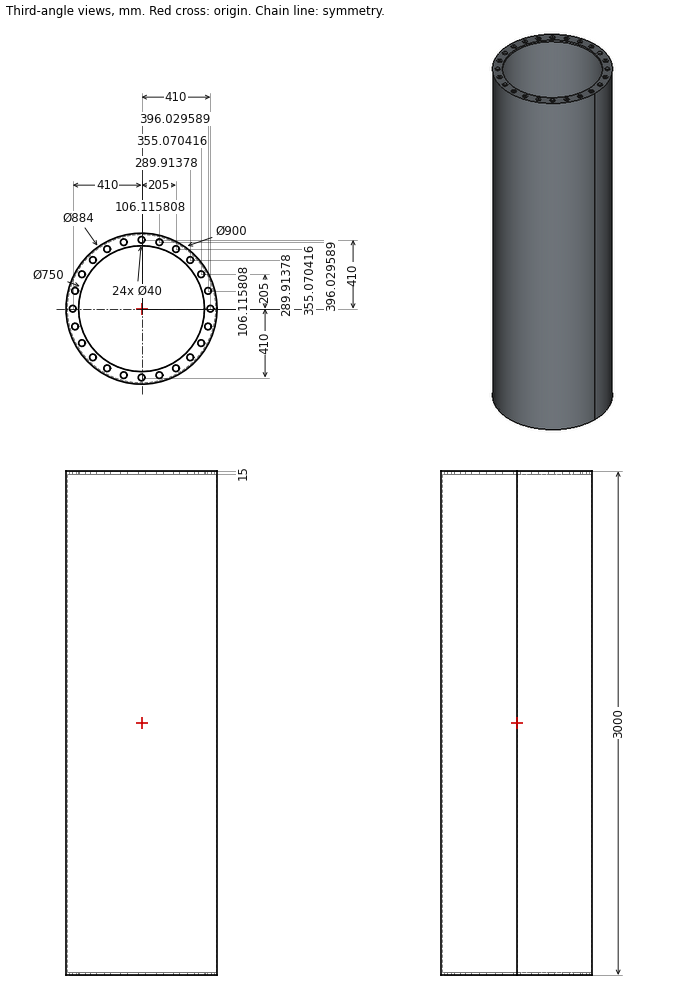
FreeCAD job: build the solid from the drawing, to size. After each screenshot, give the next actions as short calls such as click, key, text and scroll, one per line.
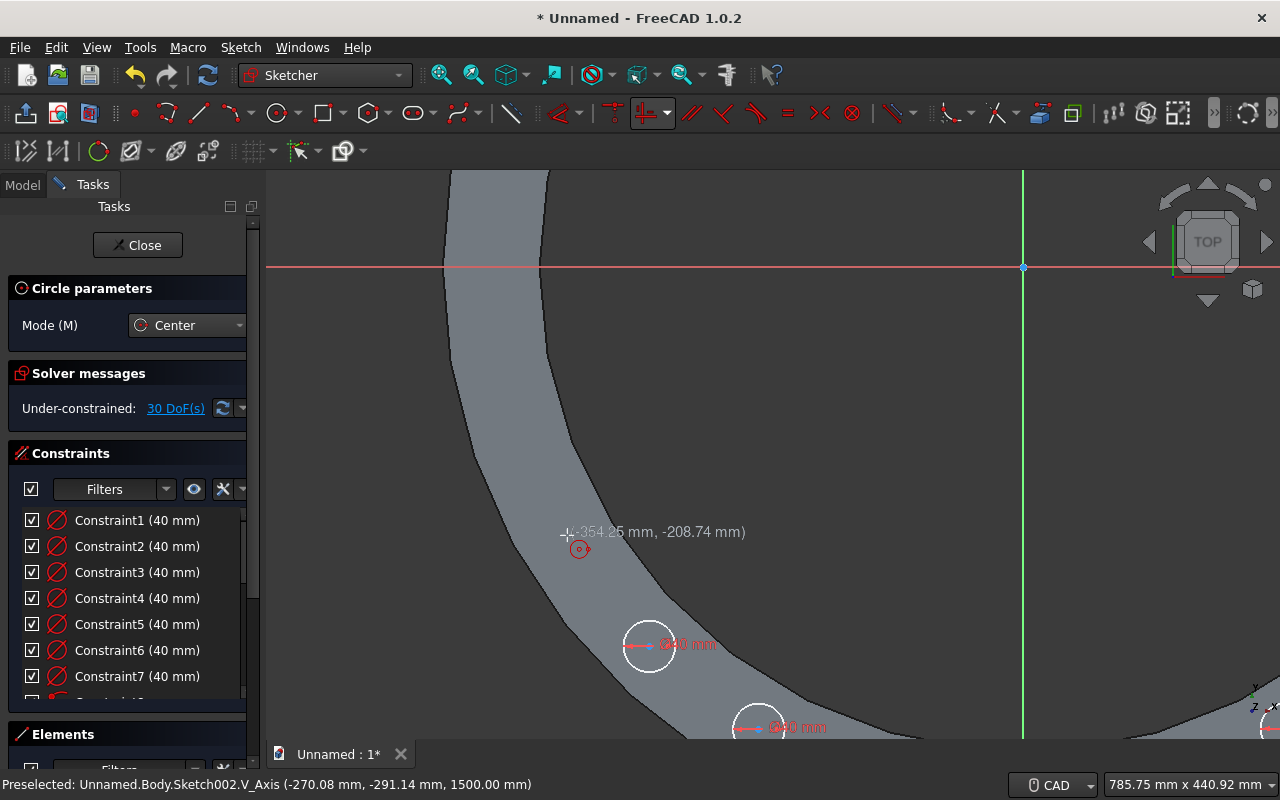
scroll(567, 535, down, 6)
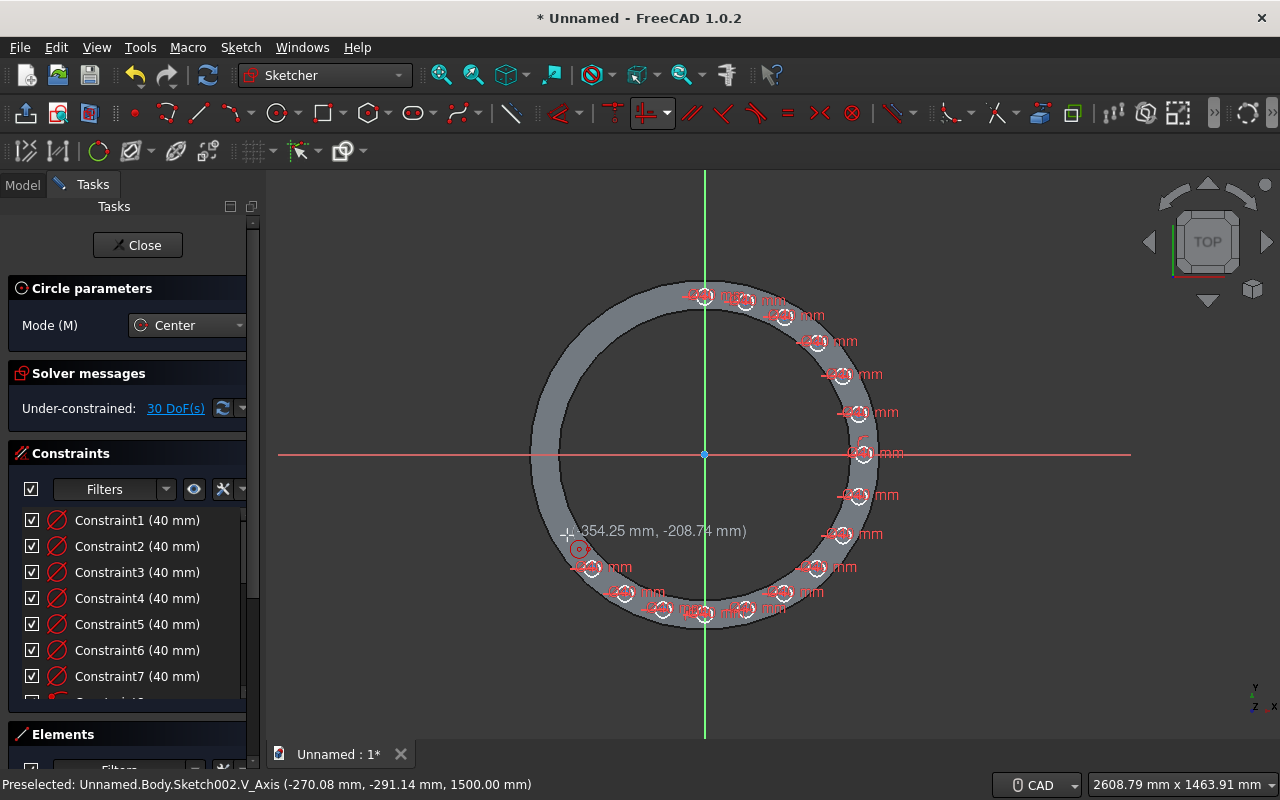
click(567, 535)
move(572, 529)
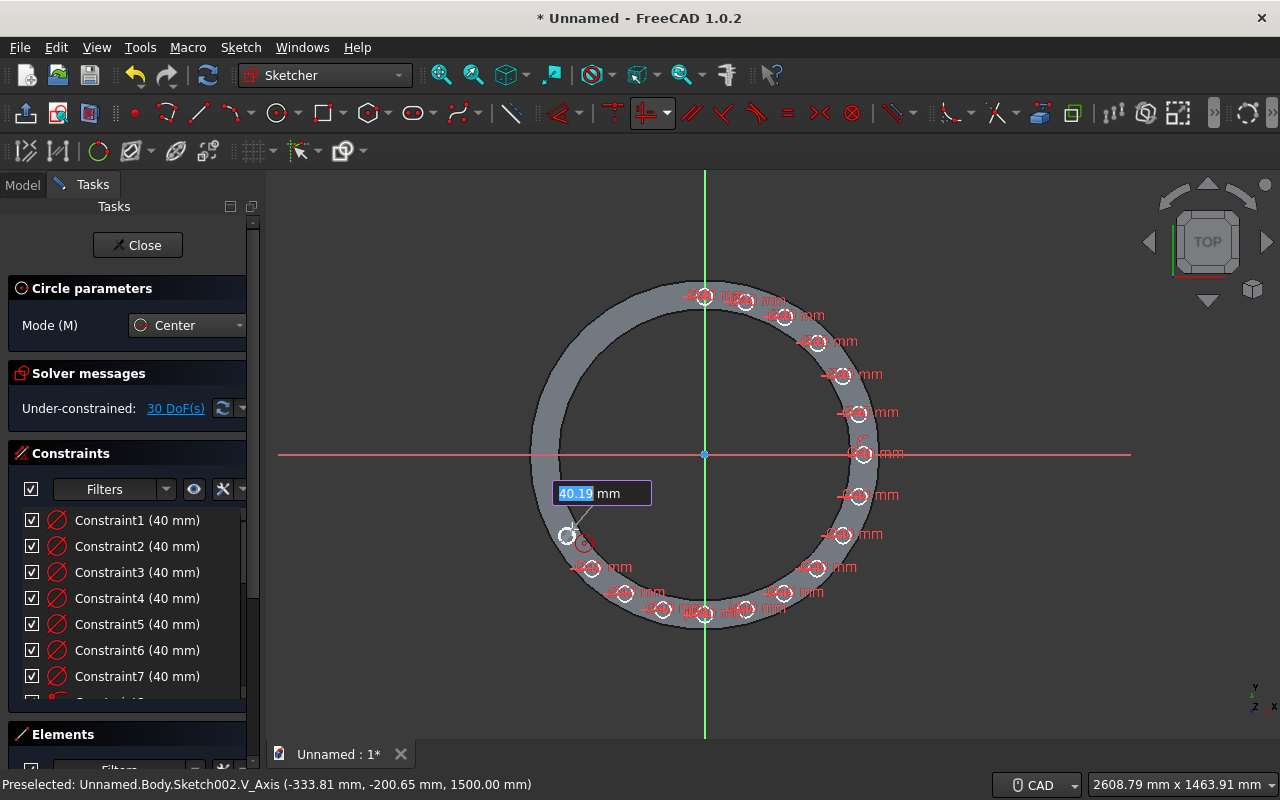
text(40)
key(Return)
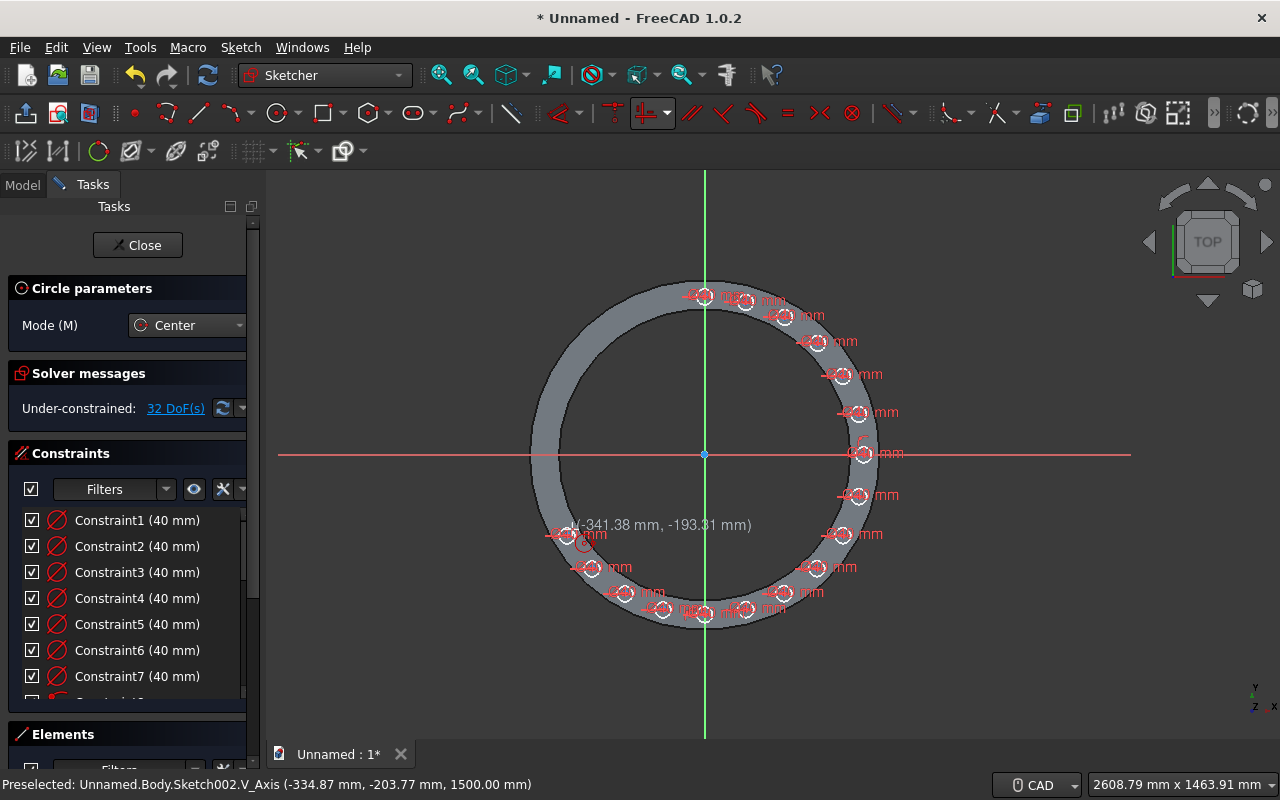
scroll(551, 496, up, 6)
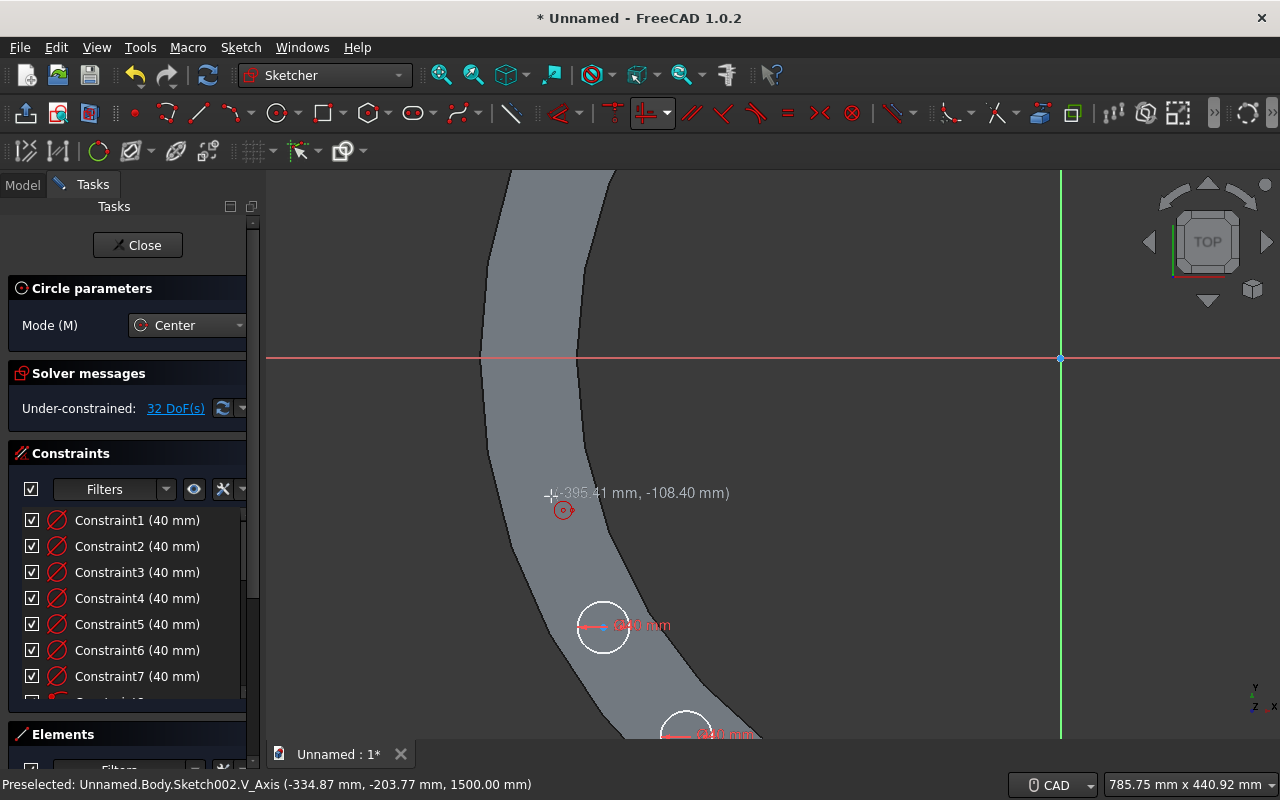
scroll(551, 496, down, 6)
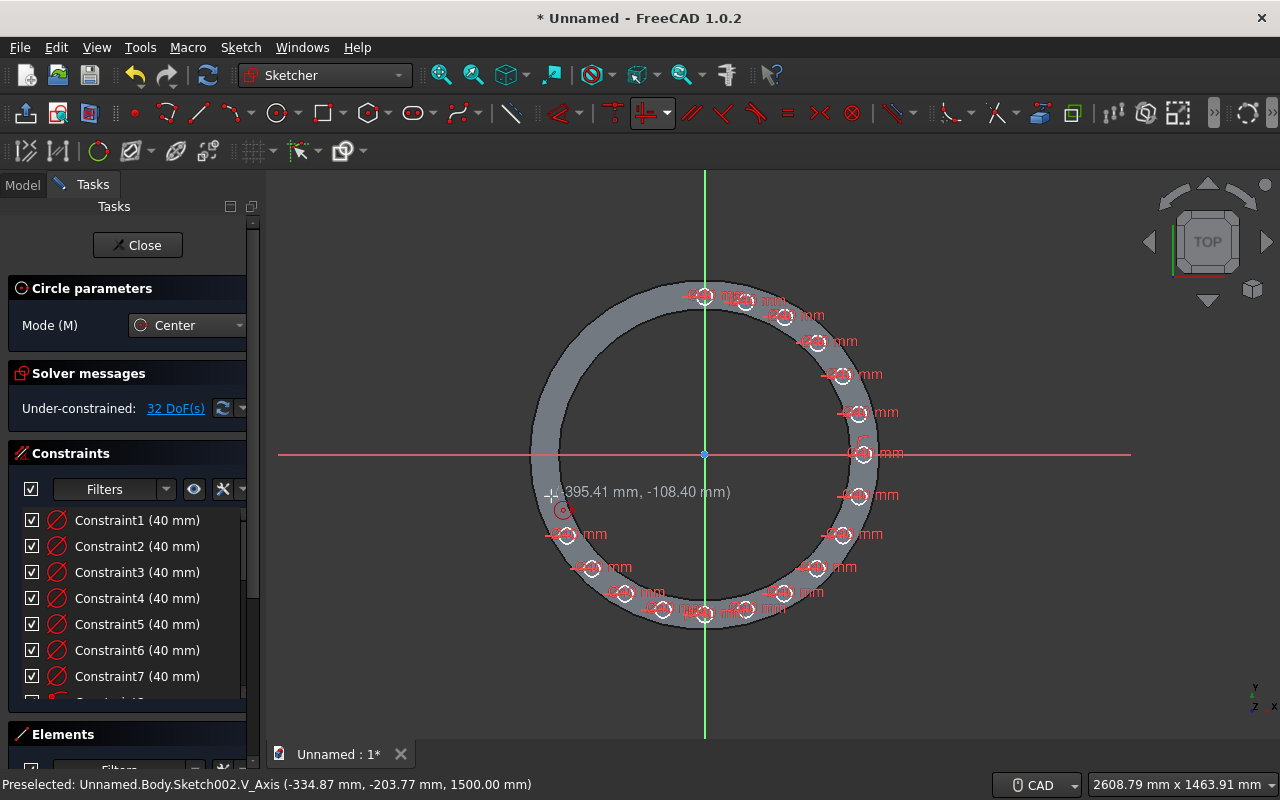
click(551, 496)
move(556, 491)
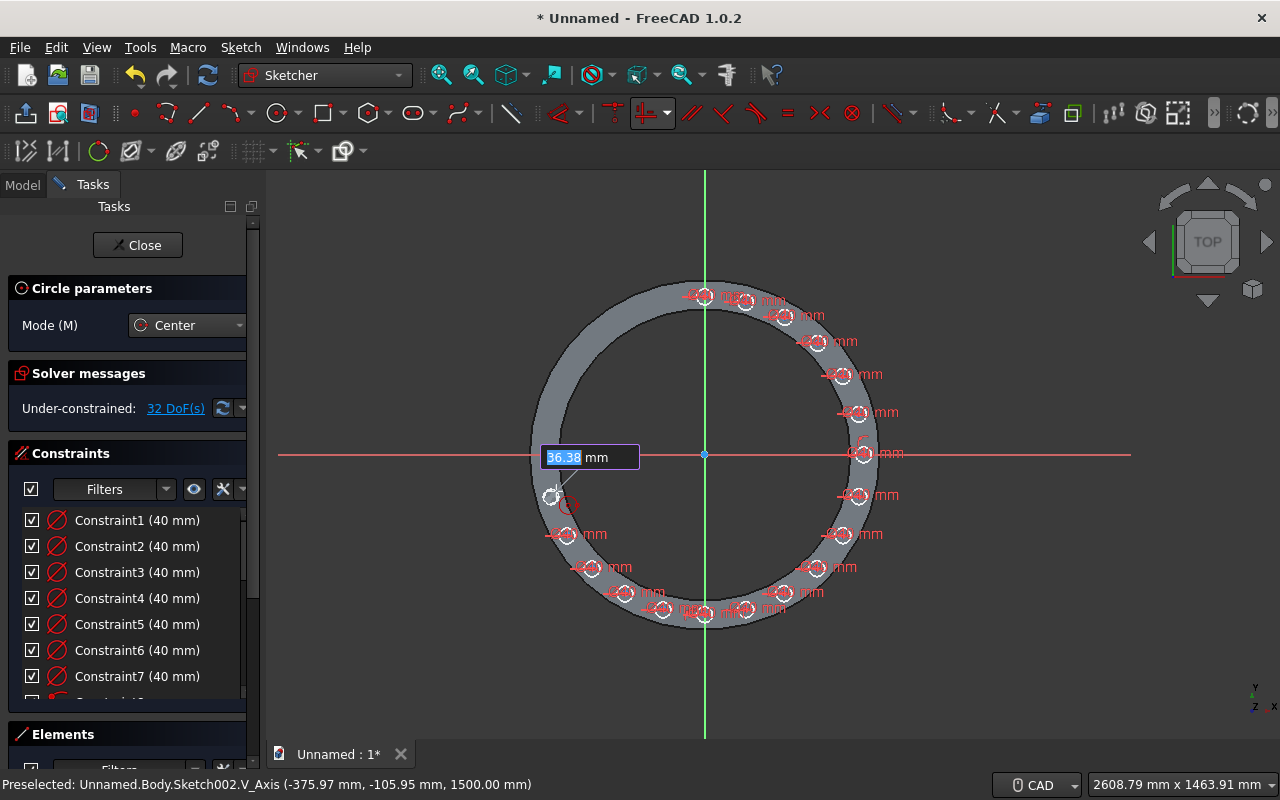
text(40)
key(Return)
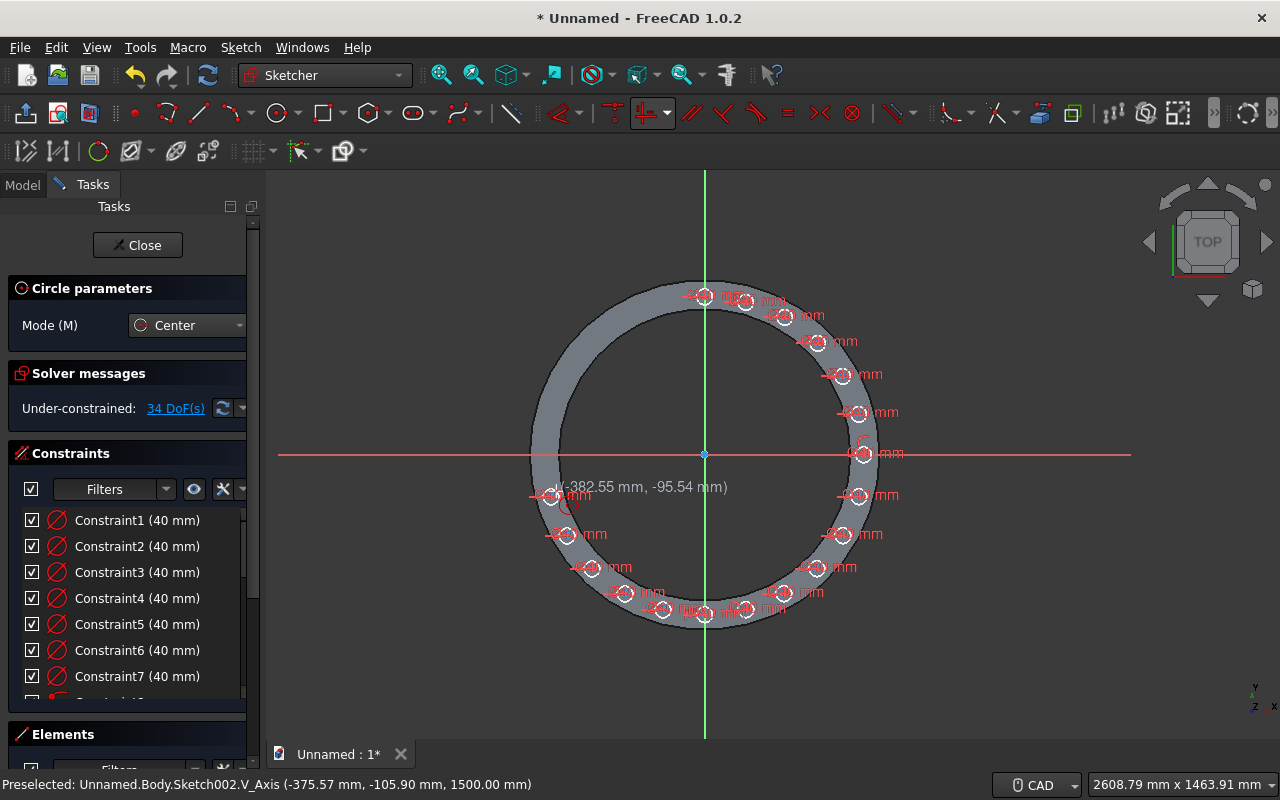
scroll(545, 455, up, 6)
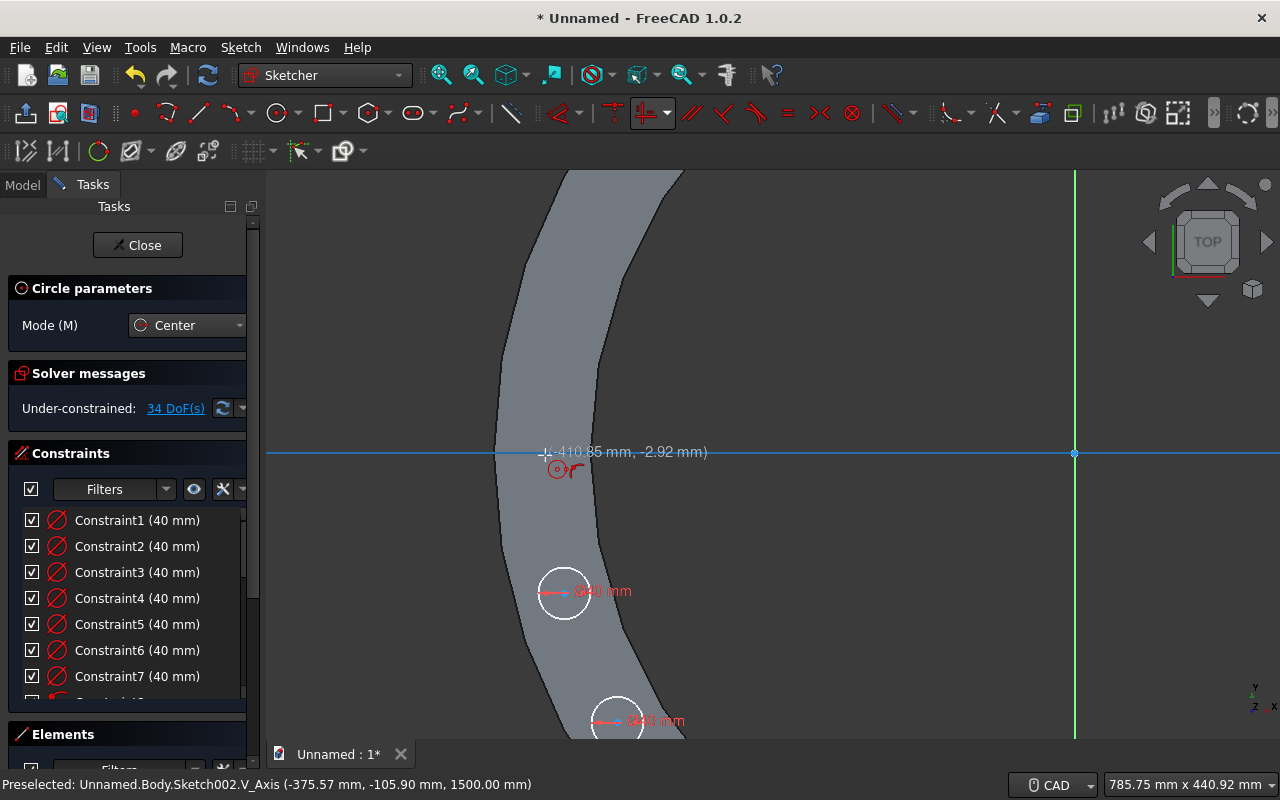
scroll(545, 455, down, 6)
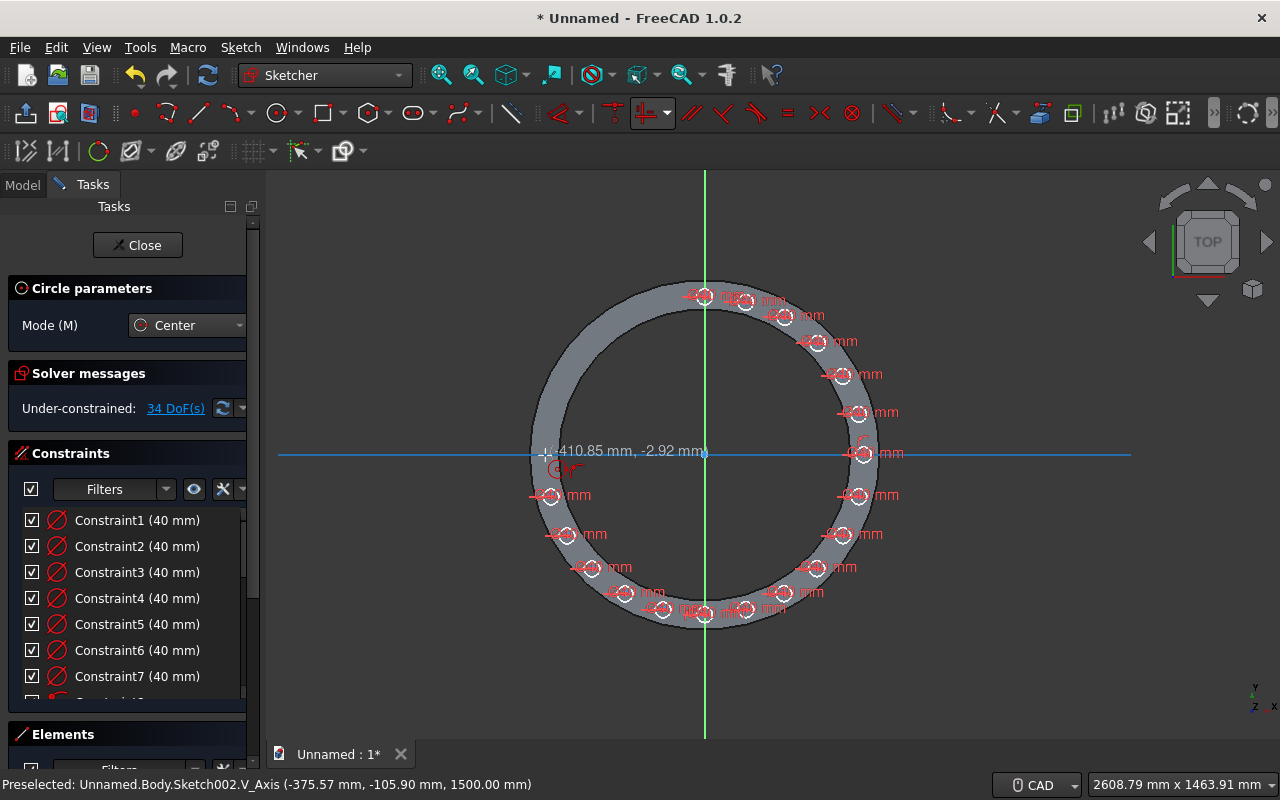
click(545, 455)